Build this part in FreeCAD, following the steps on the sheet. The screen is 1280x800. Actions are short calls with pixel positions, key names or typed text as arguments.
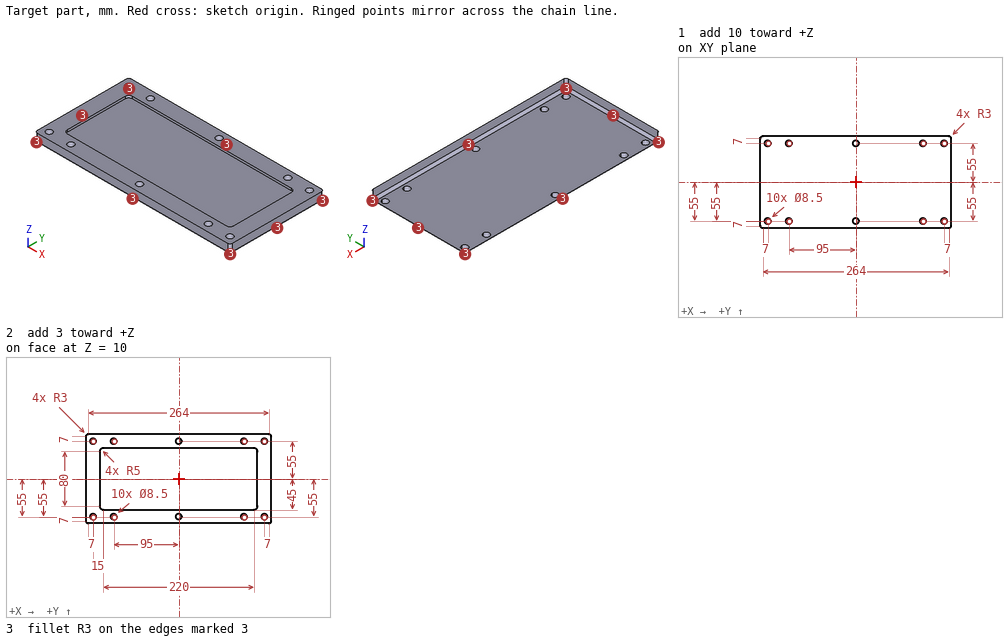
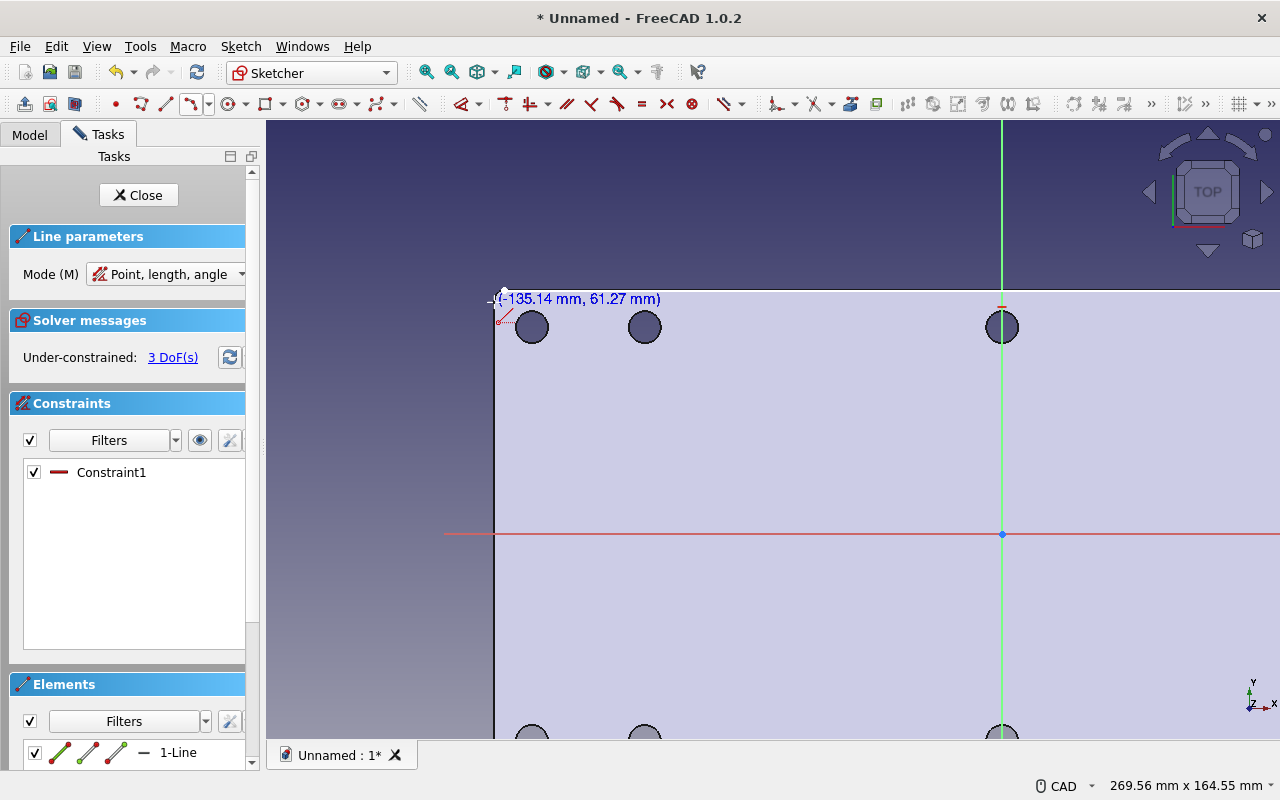
click(494, 301)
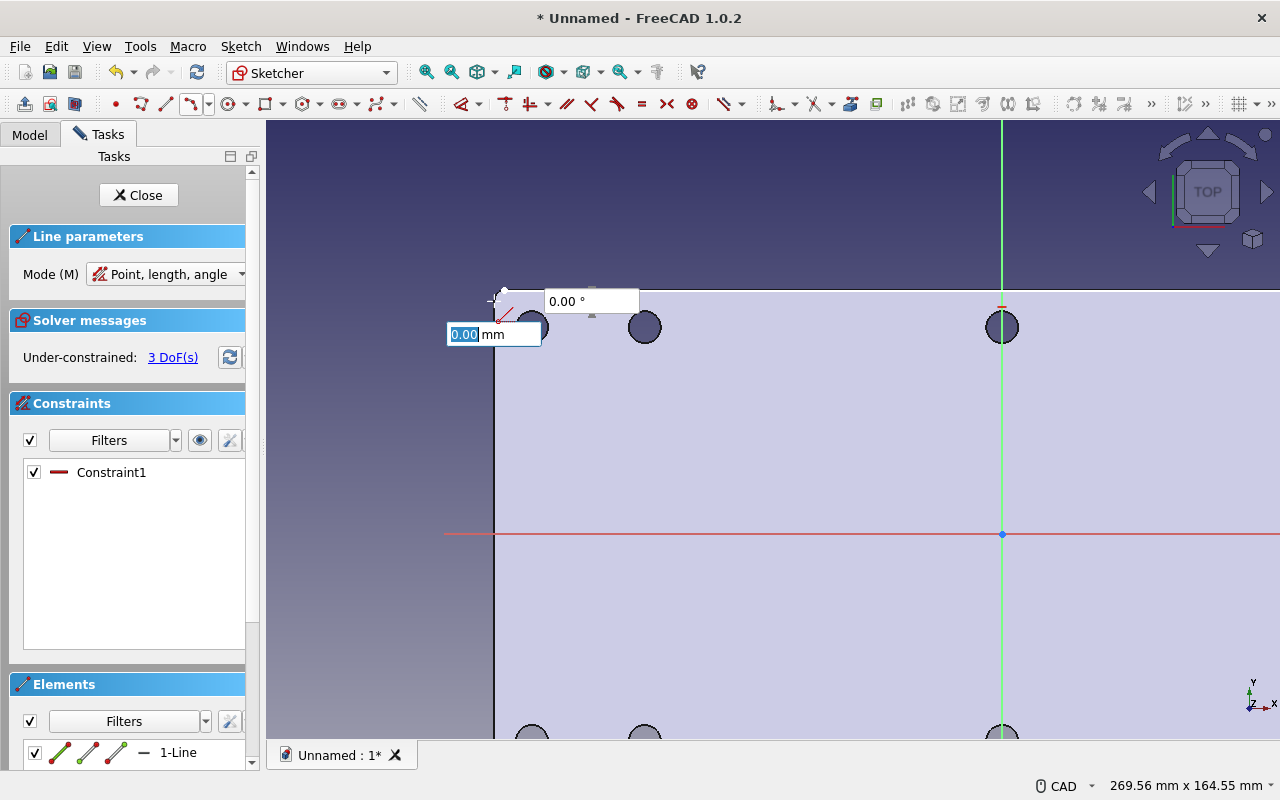
scroll(342, 302, down, 3)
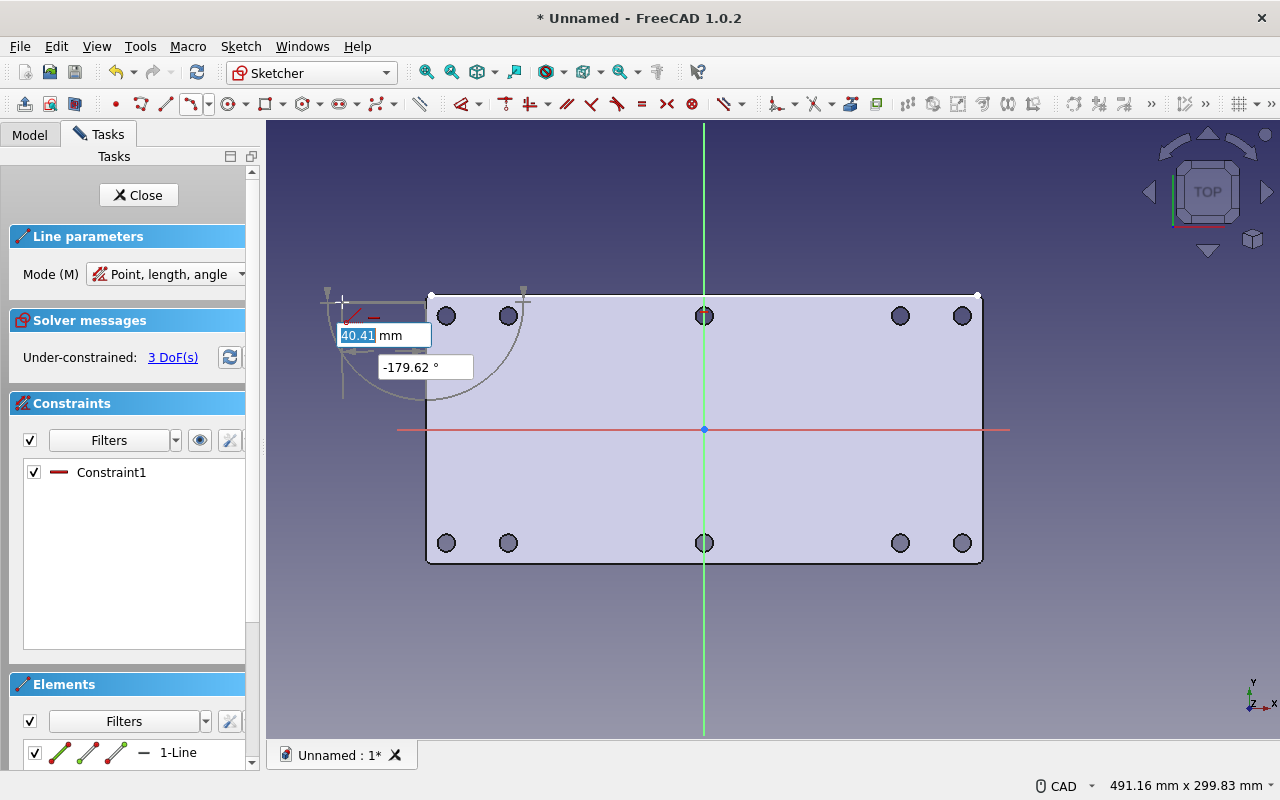
click(425, 557)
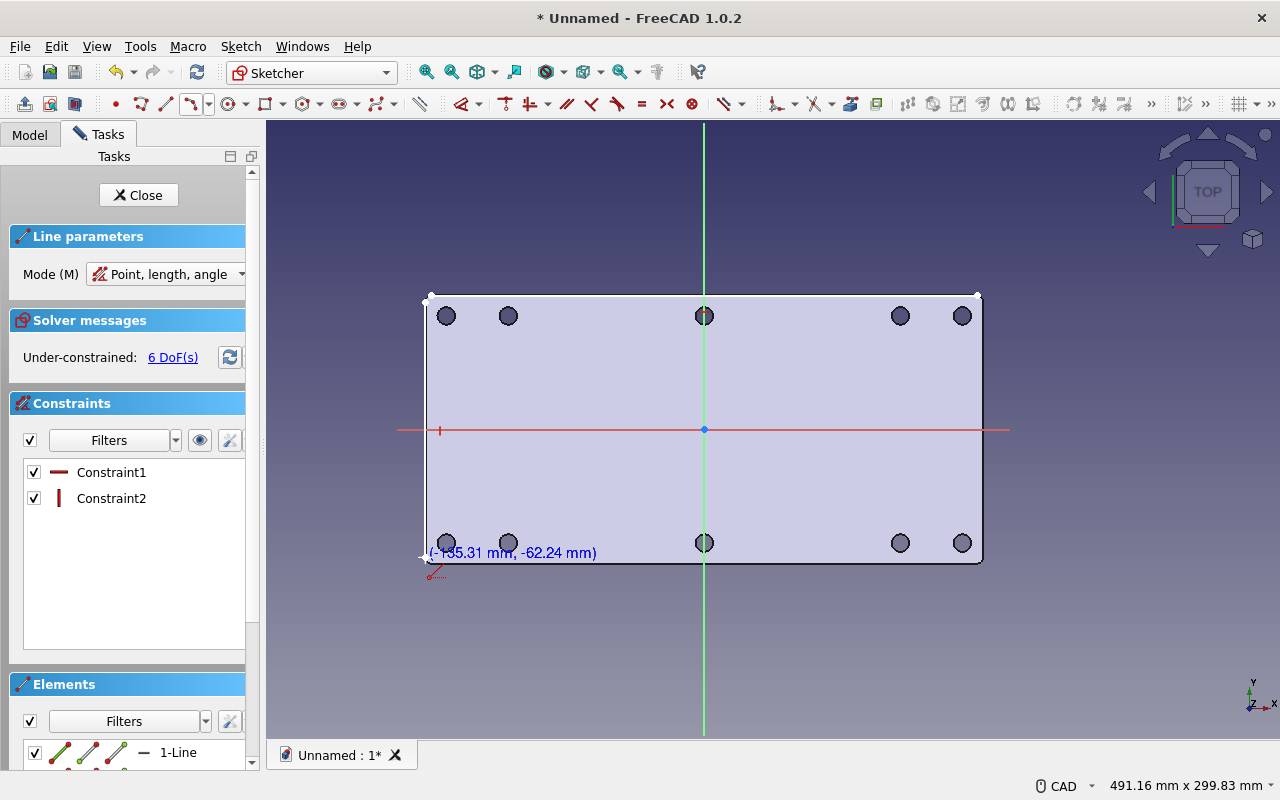
scroll(432, 564, up, 3)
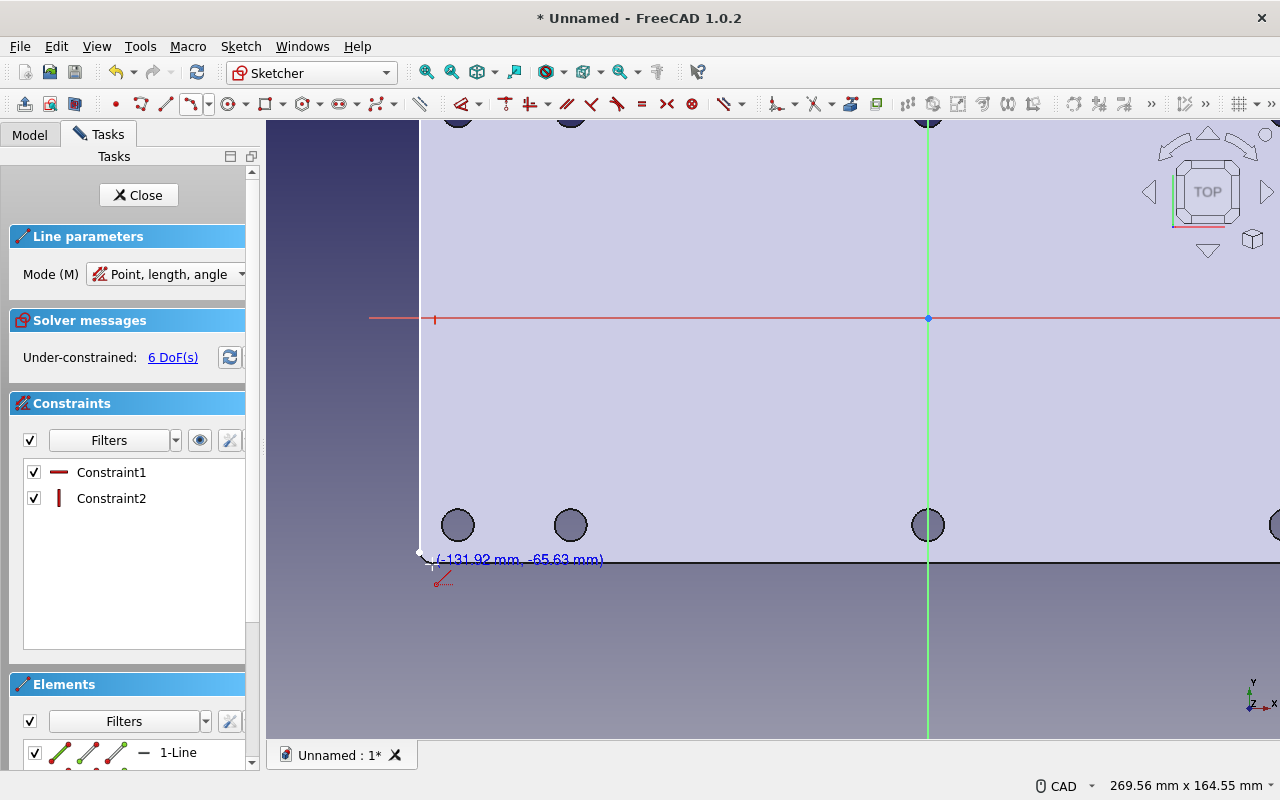
click(432, 563)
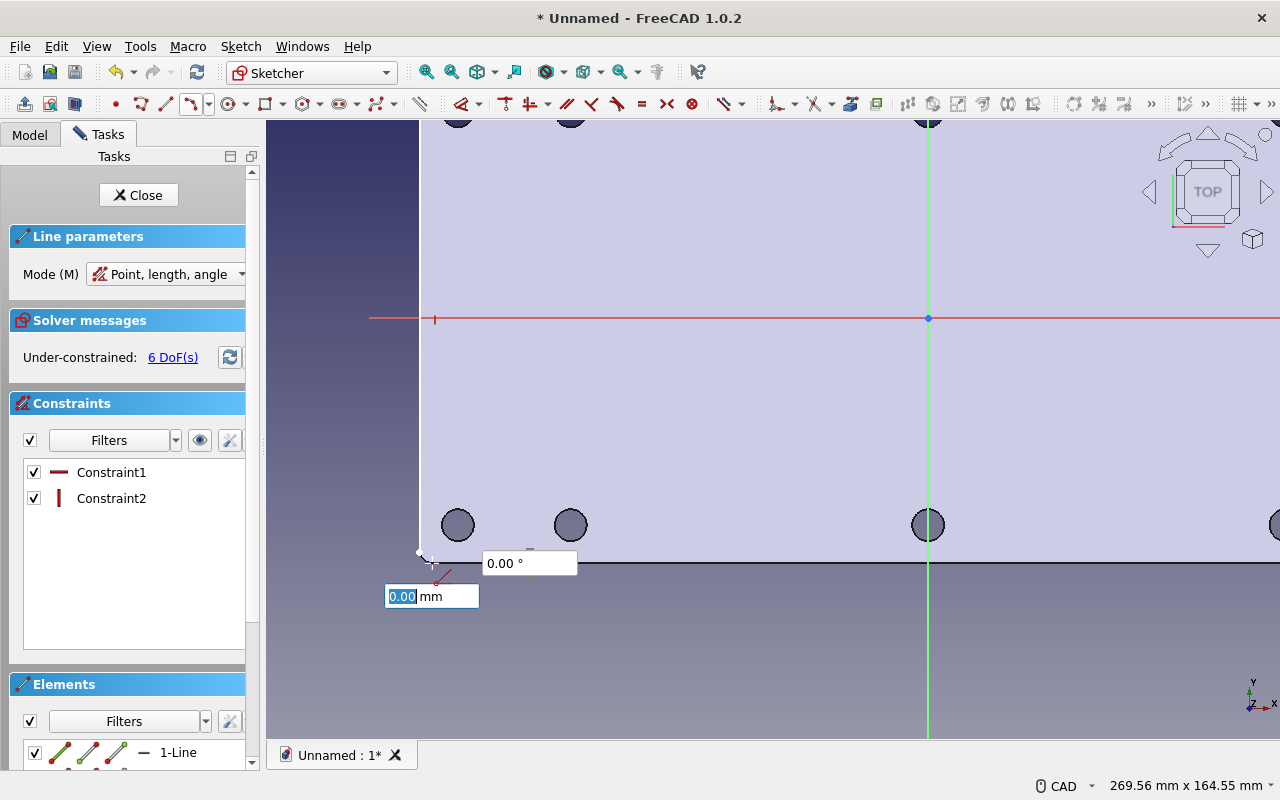
scroll(432, 565, down, 3)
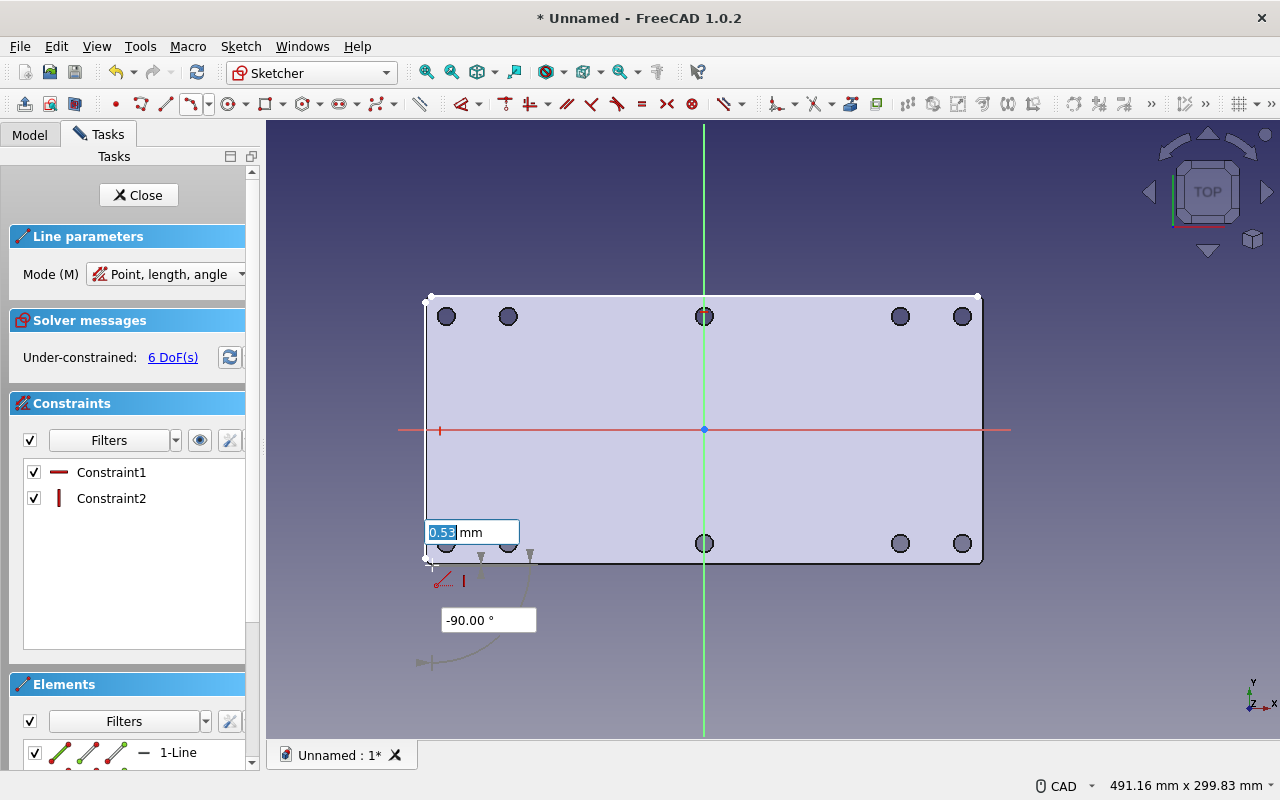
click(977, 564)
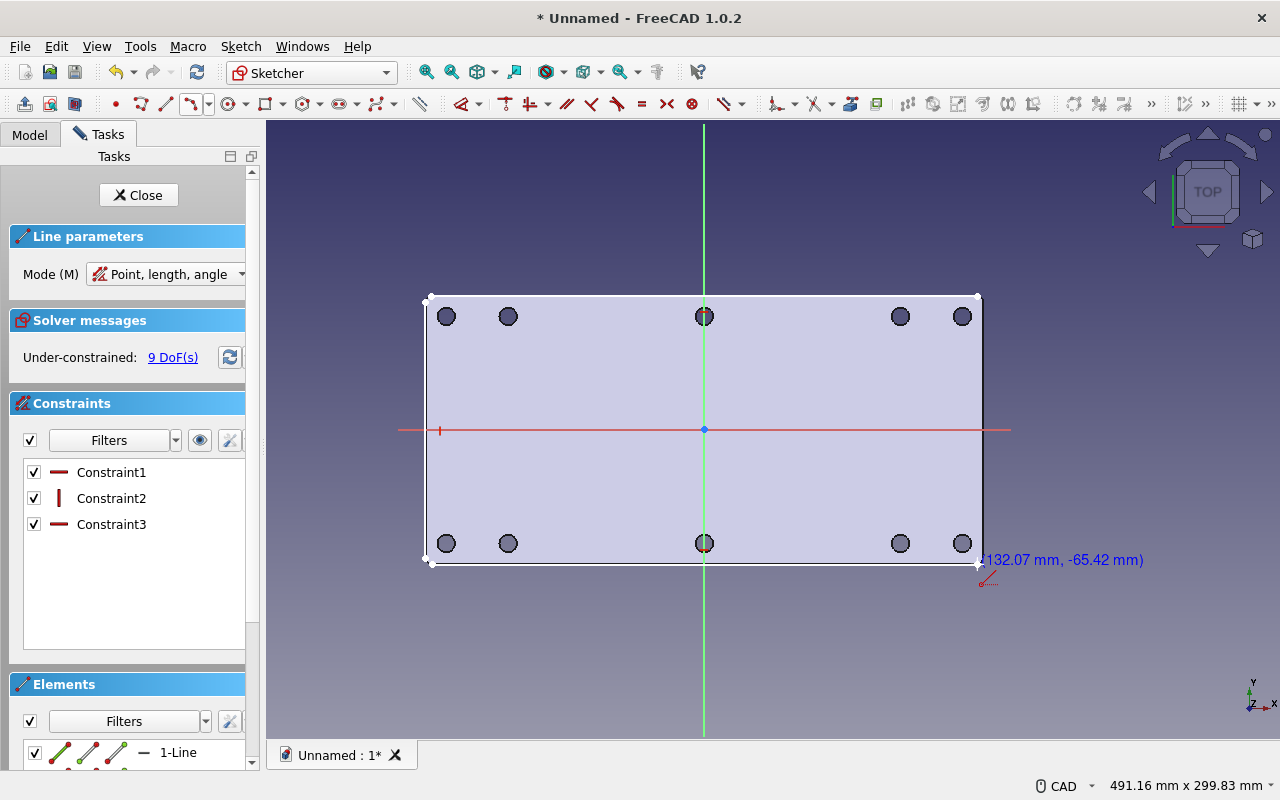
scroll(983, 558, up, 3)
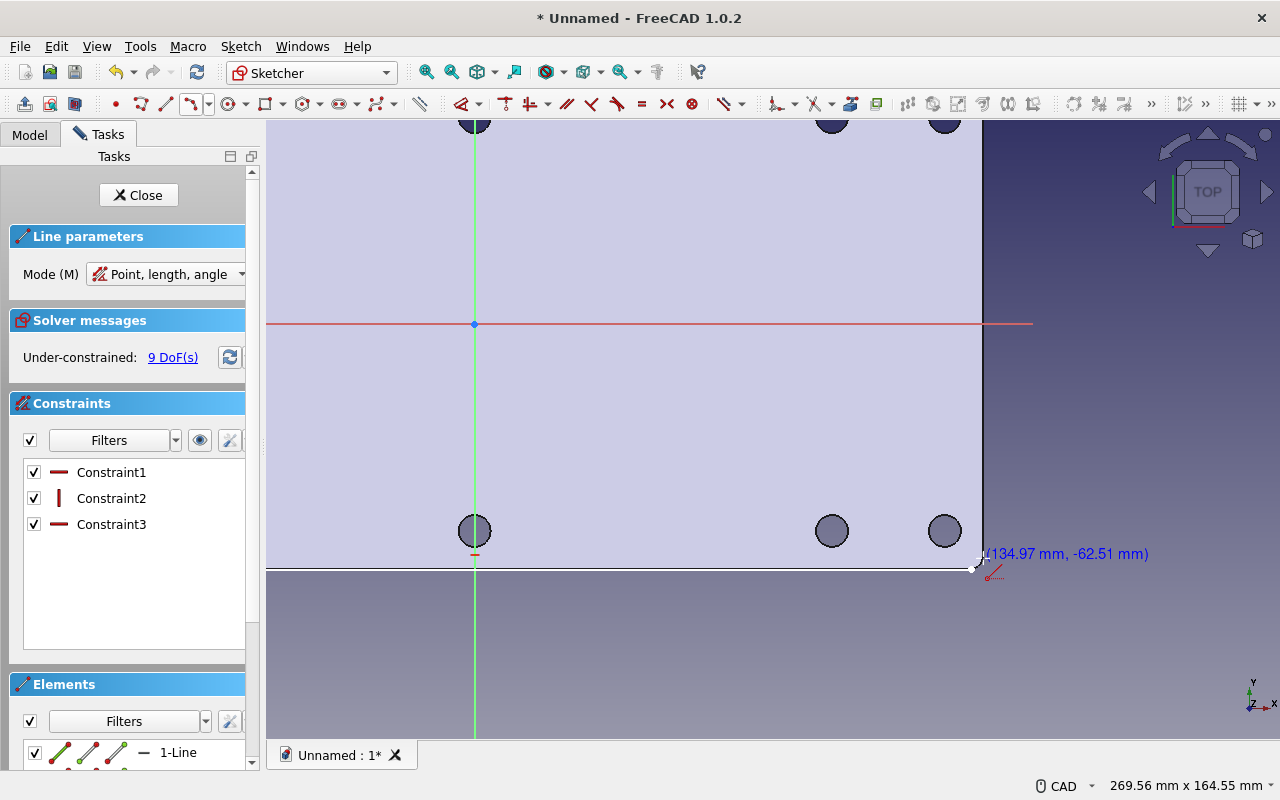
click(983, 557)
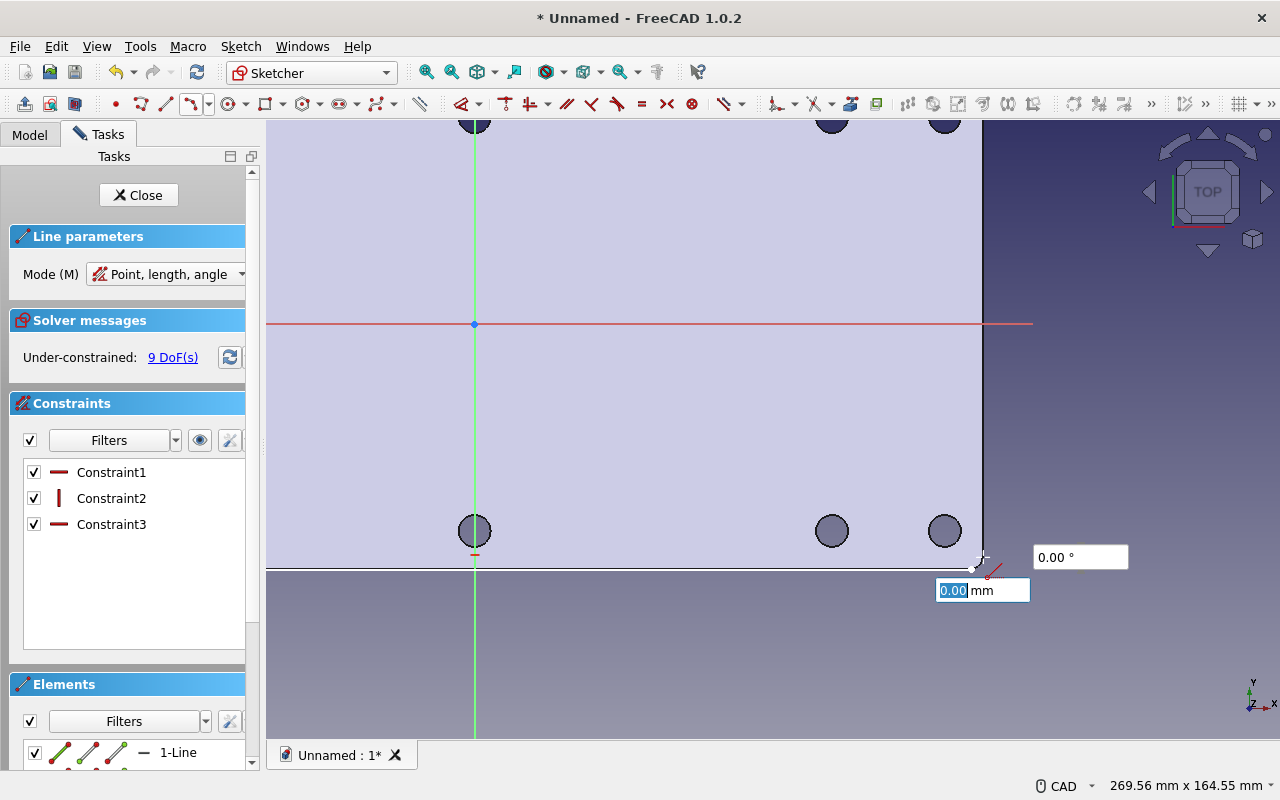
scroll(984, 558, down, 3)